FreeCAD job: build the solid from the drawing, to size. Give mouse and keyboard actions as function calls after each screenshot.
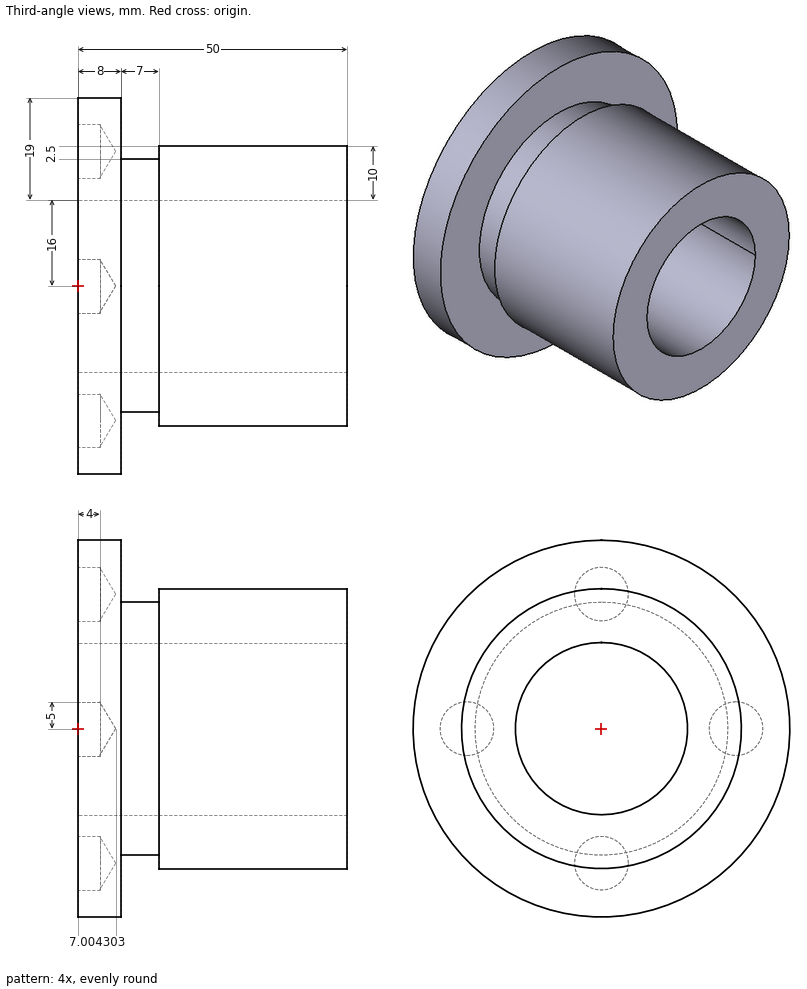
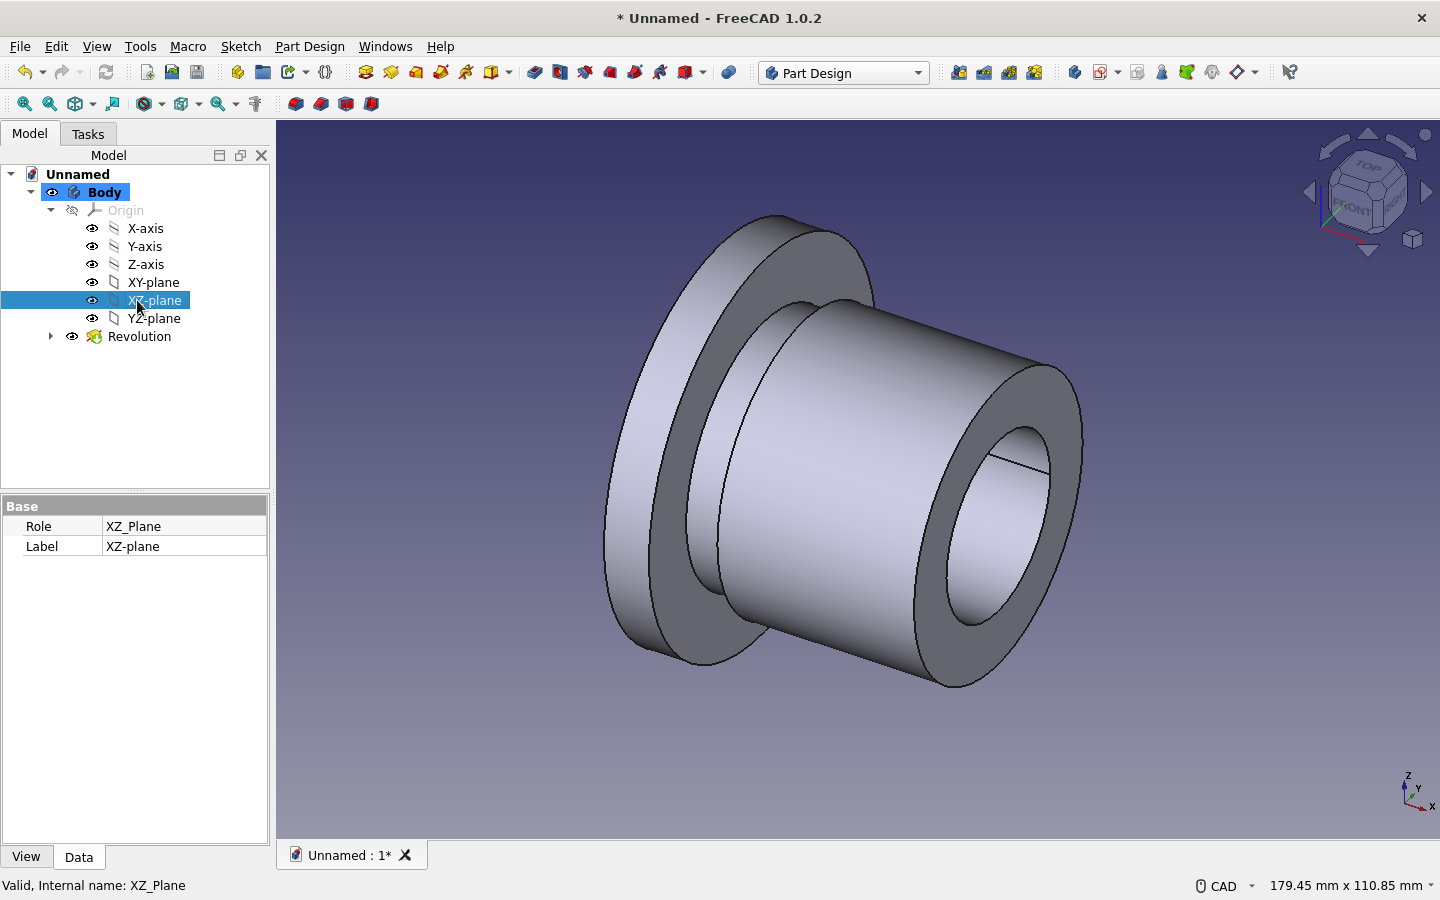
click(1236, 72)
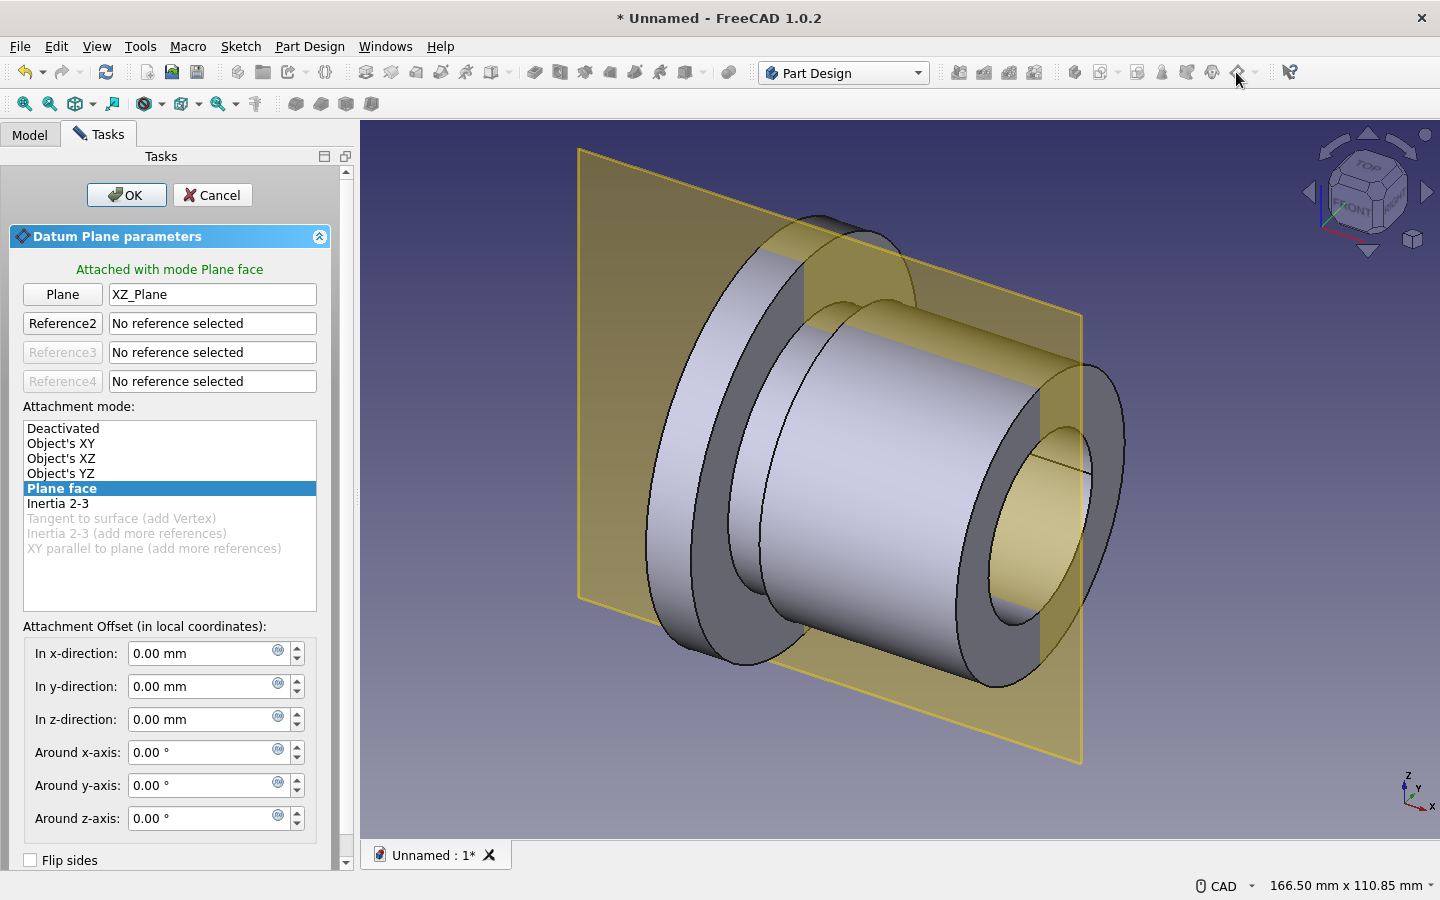
triple_click(210, 720)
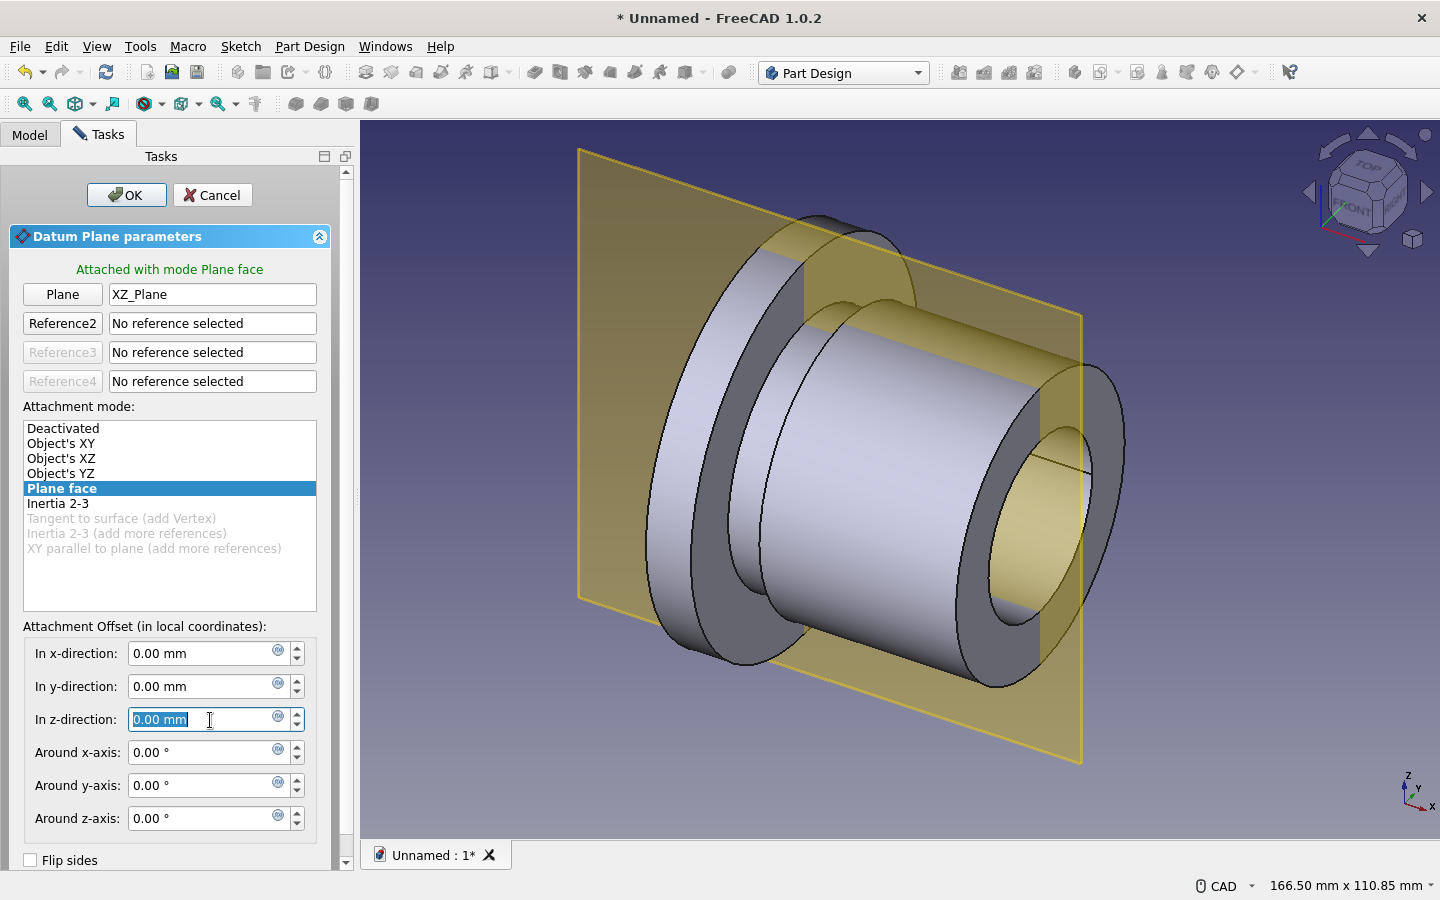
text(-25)
key(Tab)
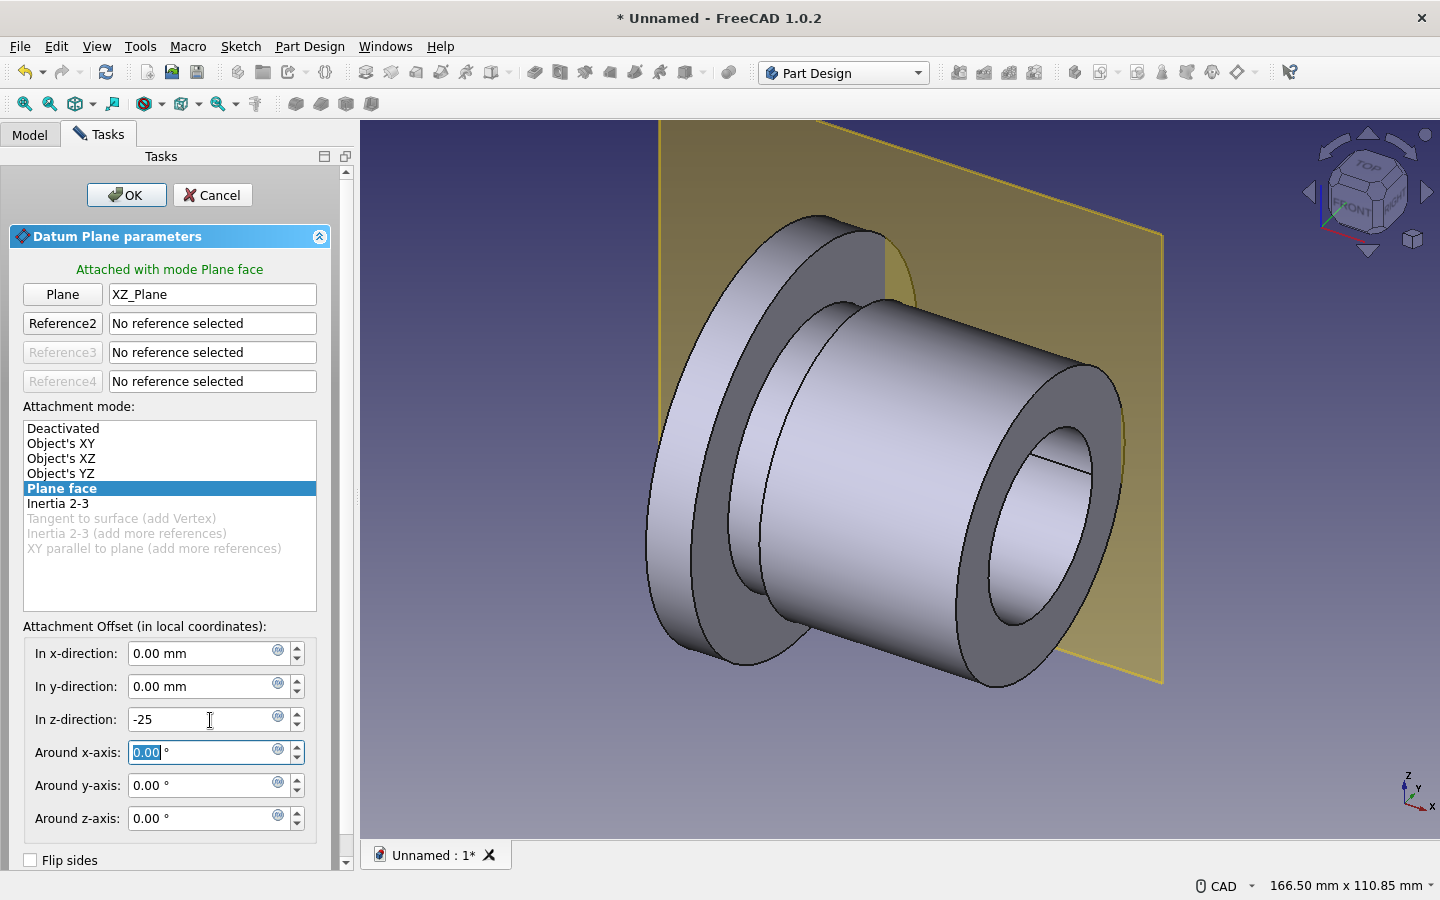
click(127, 195)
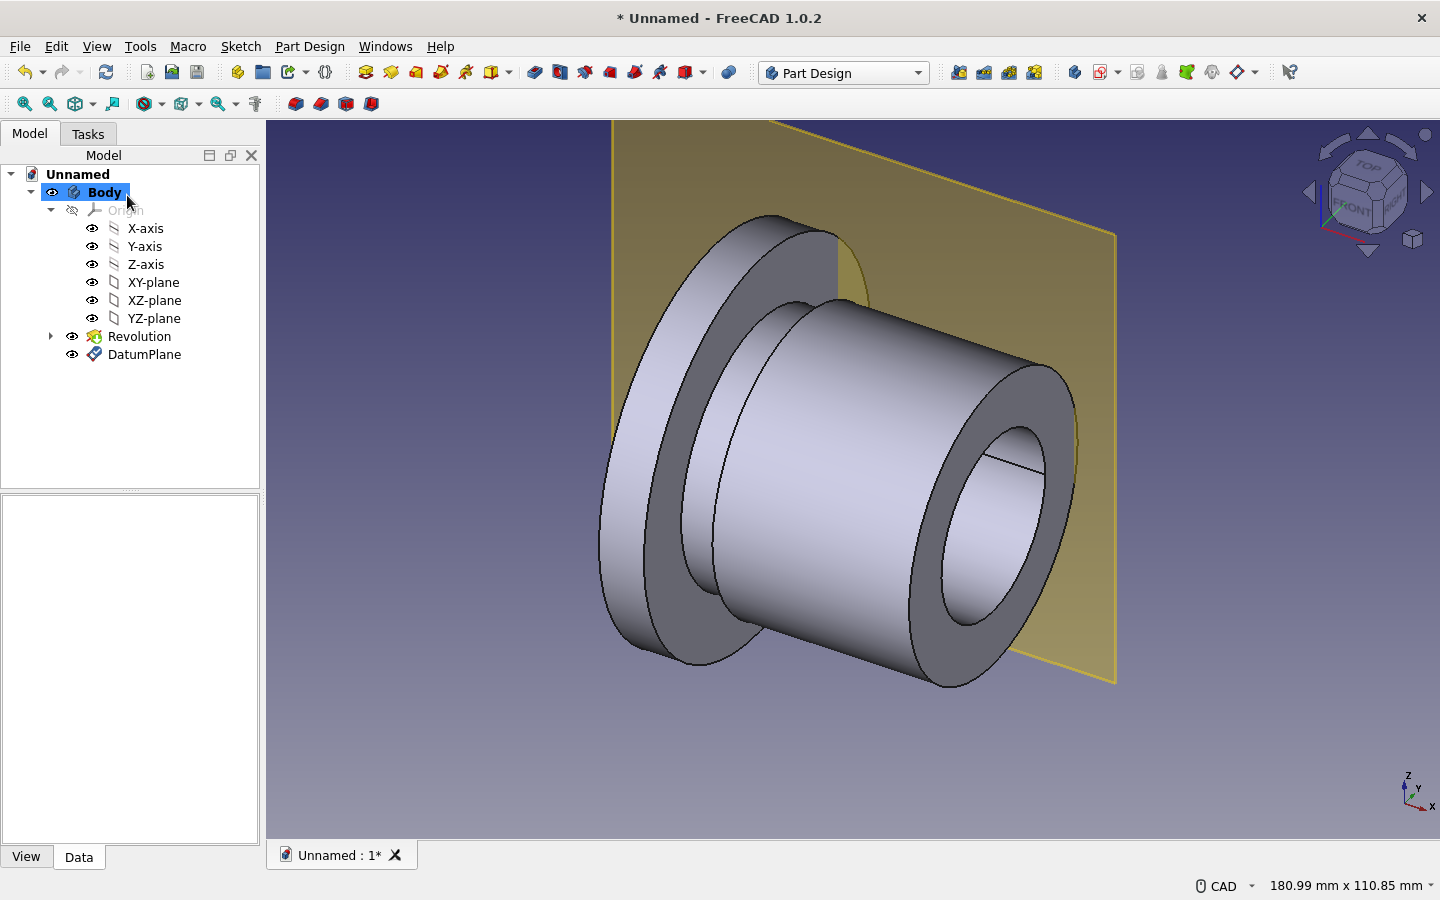
click(117, 354)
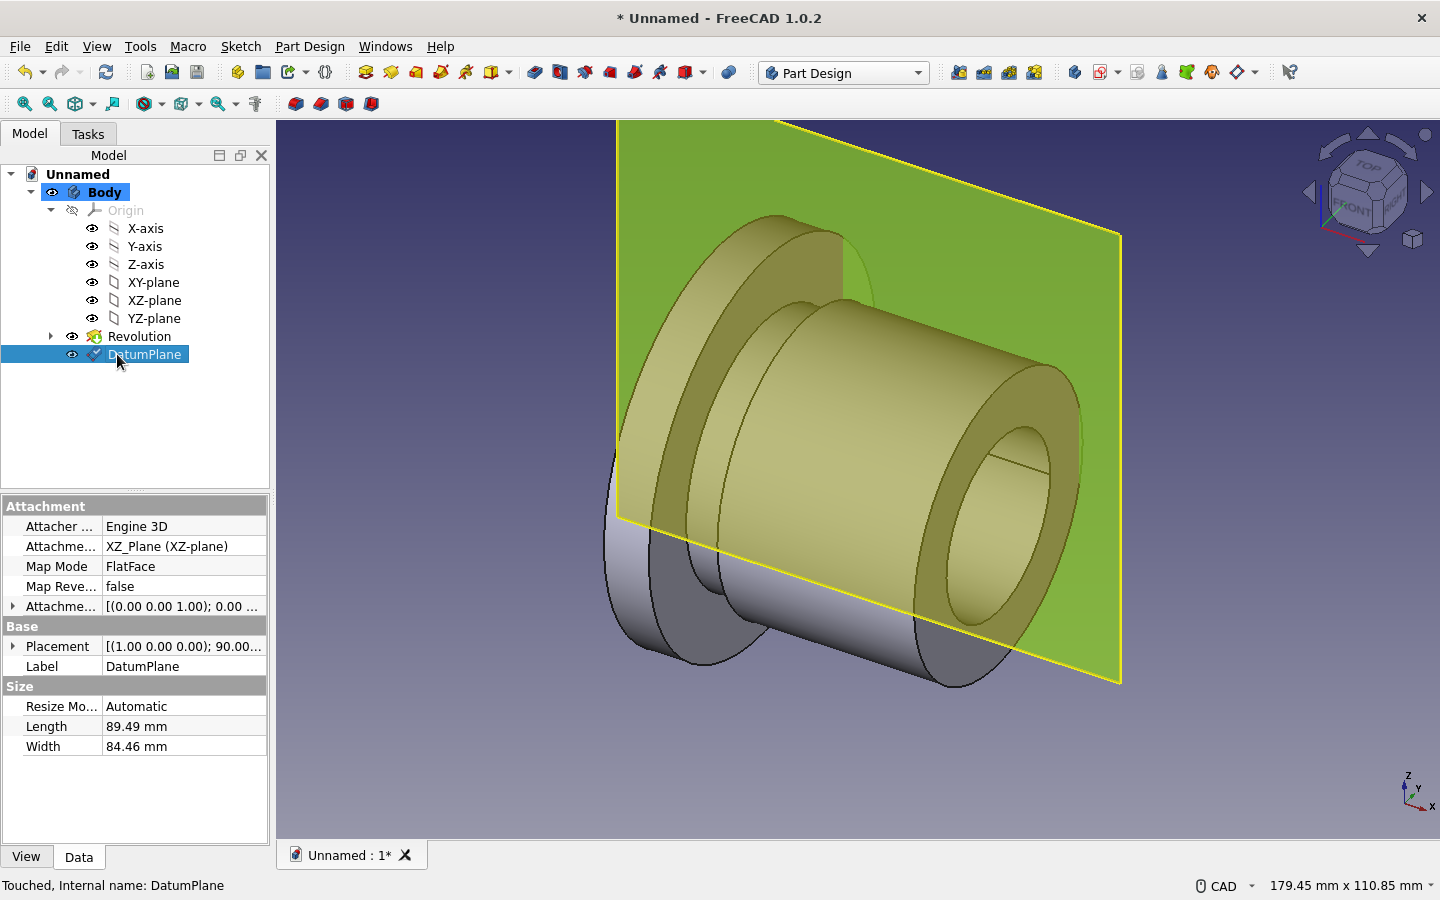
click(1100, 72)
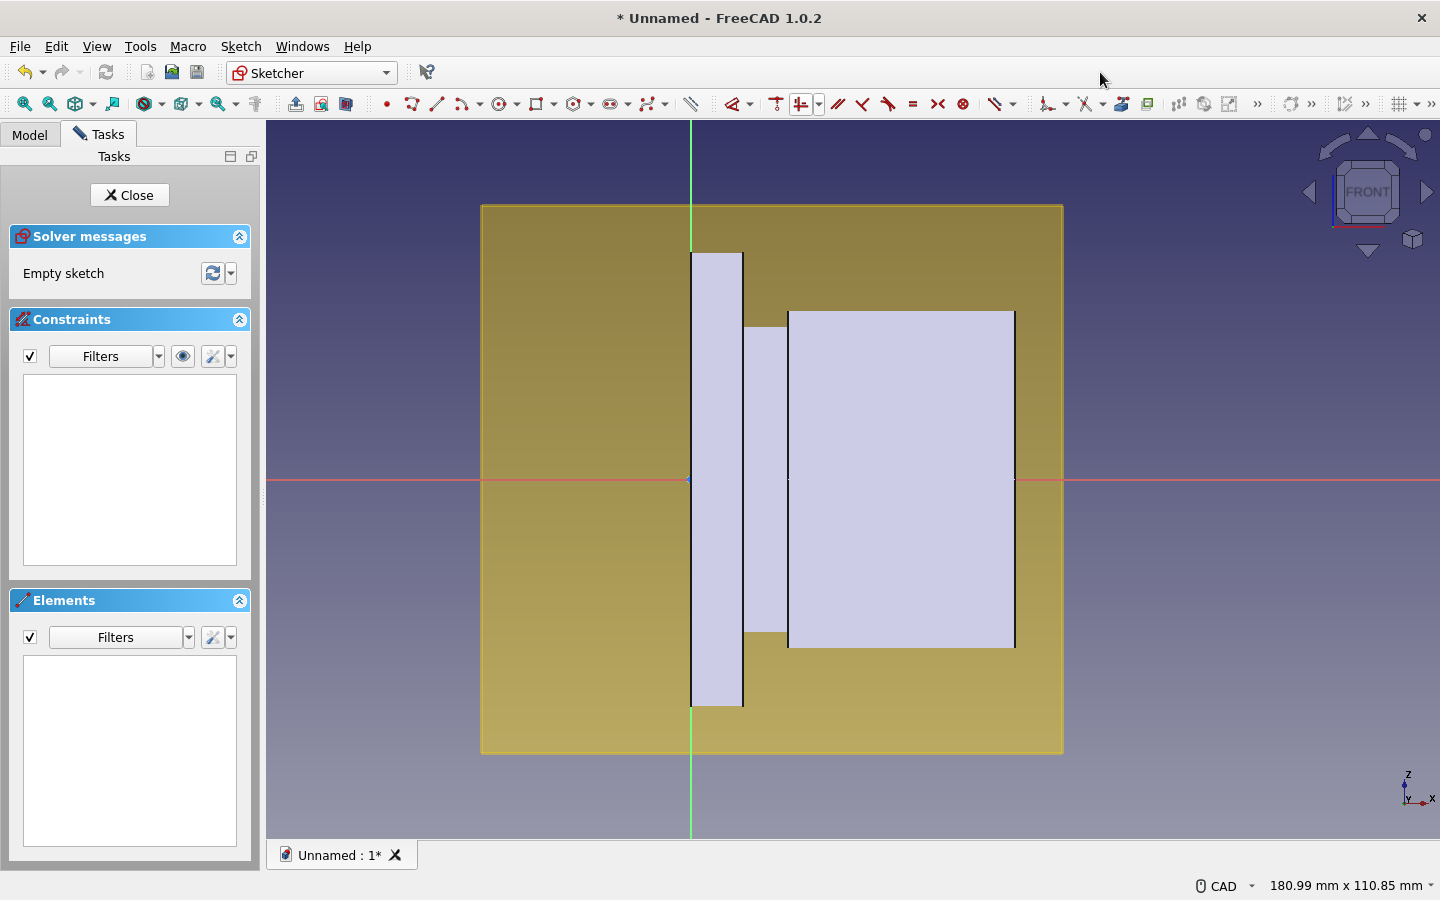
key(q)
key(s)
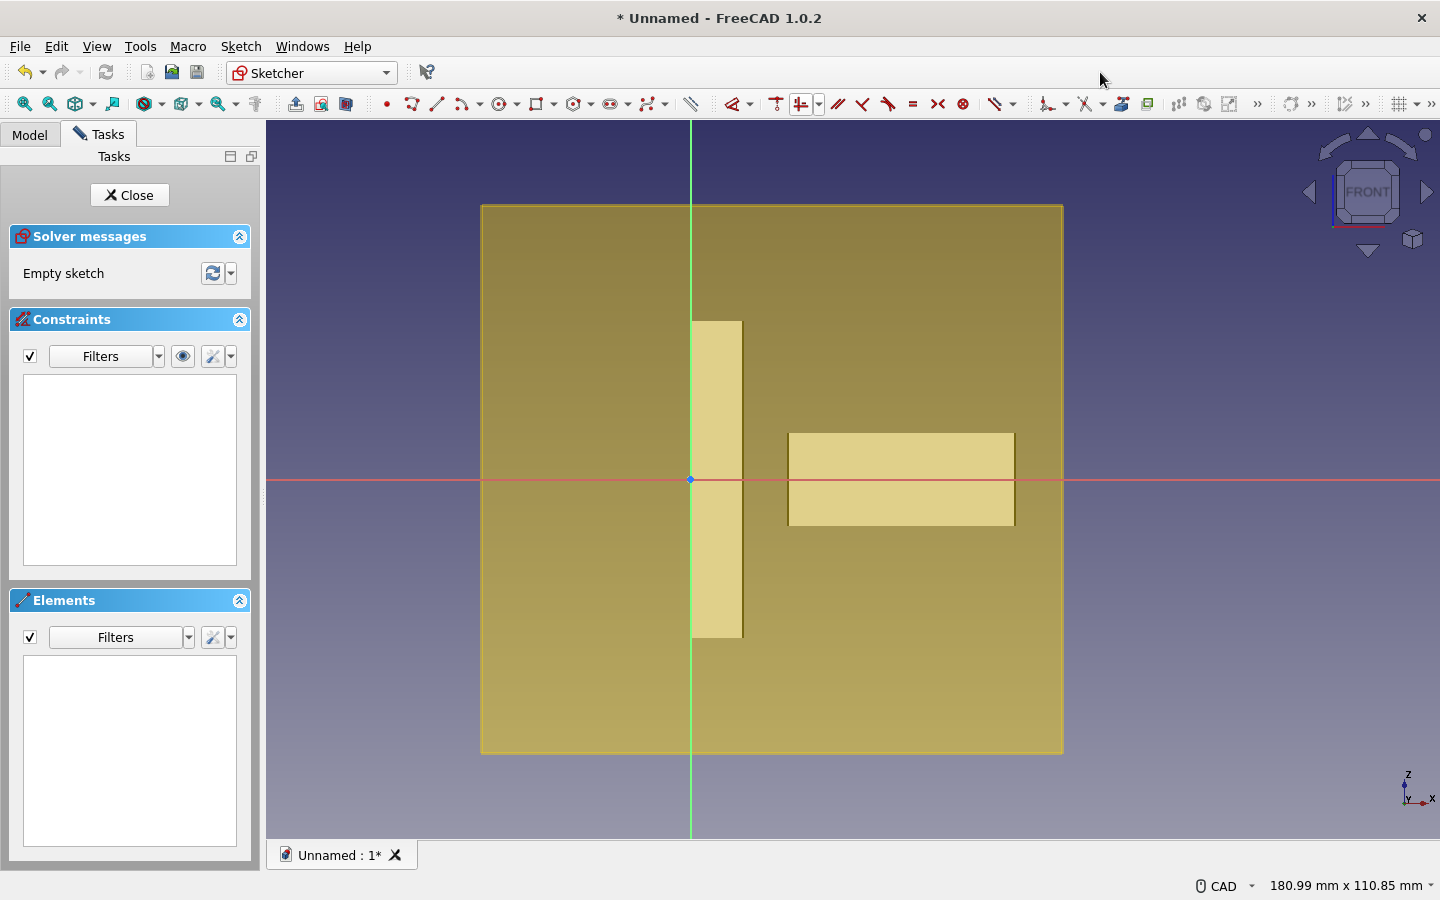
scroll(708, 462, up, 13)